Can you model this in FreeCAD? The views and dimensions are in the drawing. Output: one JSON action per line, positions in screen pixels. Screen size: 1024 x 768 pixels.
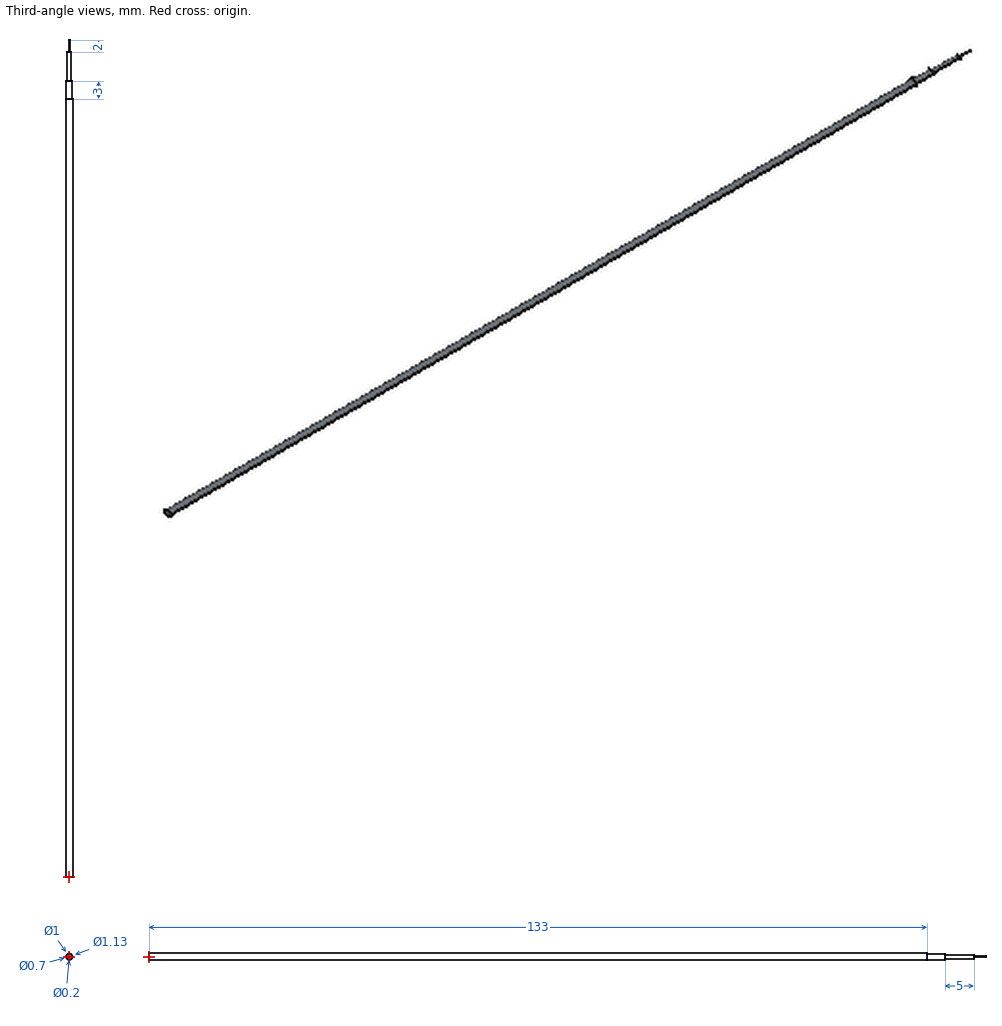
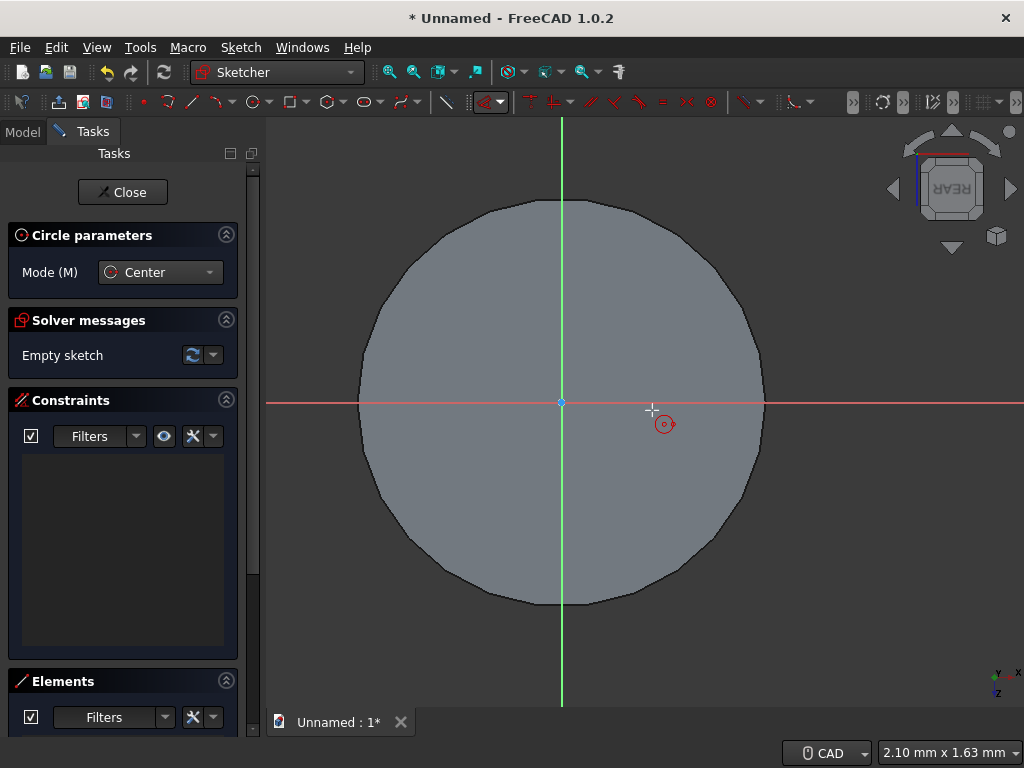
{"action": "left_click", "coordinate": [562, 403]}
{"action": "left_click", "coordinate": [689, 275]}
{"action": "key", "text": "Escape"}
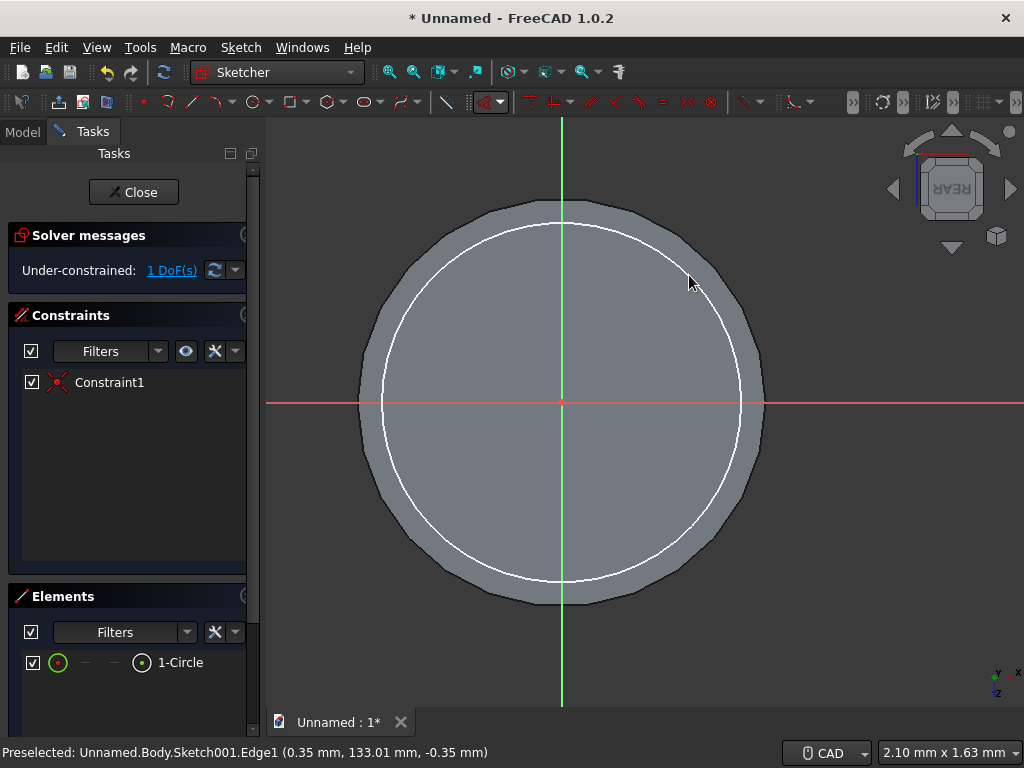
{"action": "left_click", "coordinate": [688, 275]}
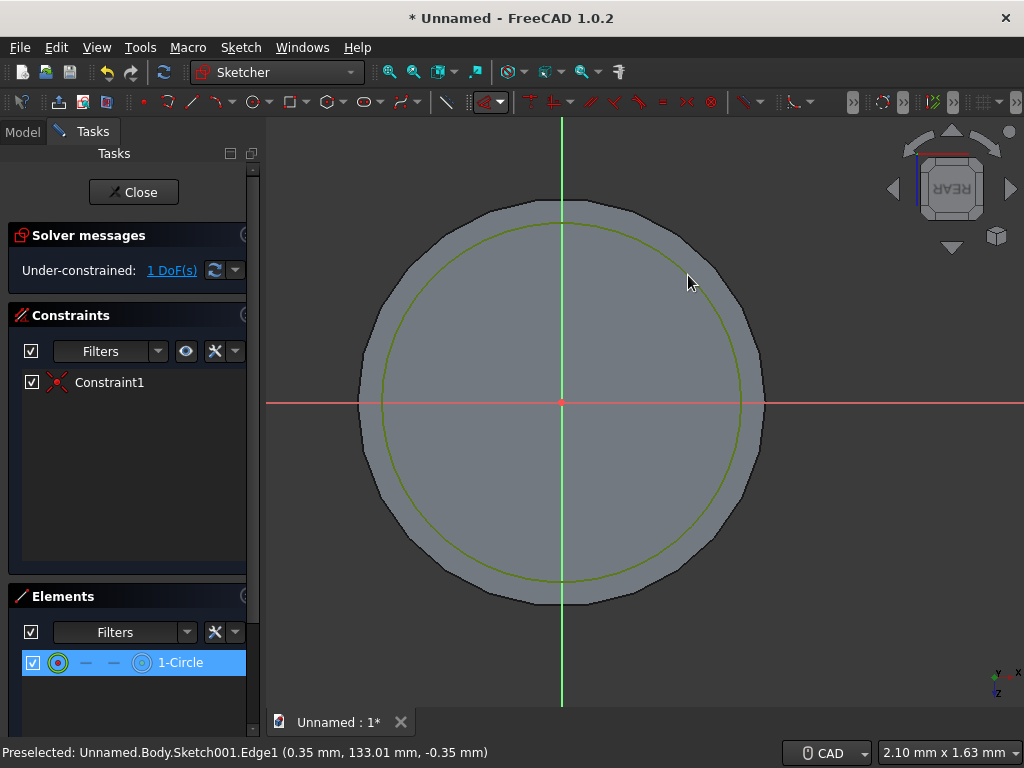
{"action": "left_click", "coordinate": [502, 102]}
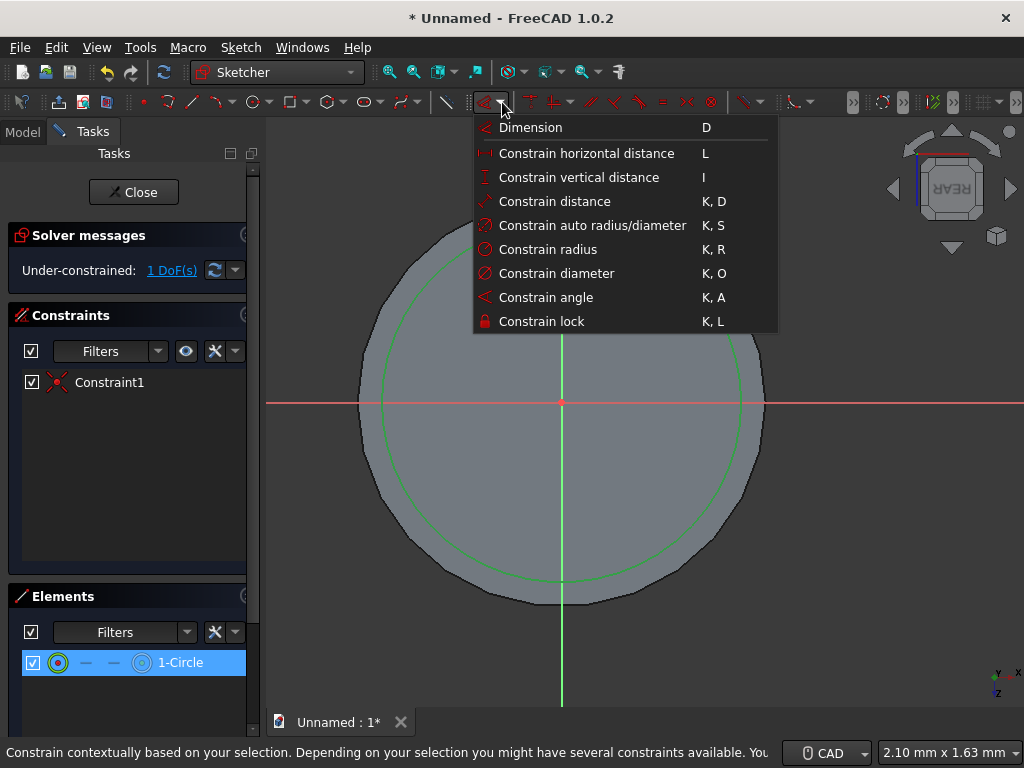
{"action": "left_click", "coordinate": [626, 273]}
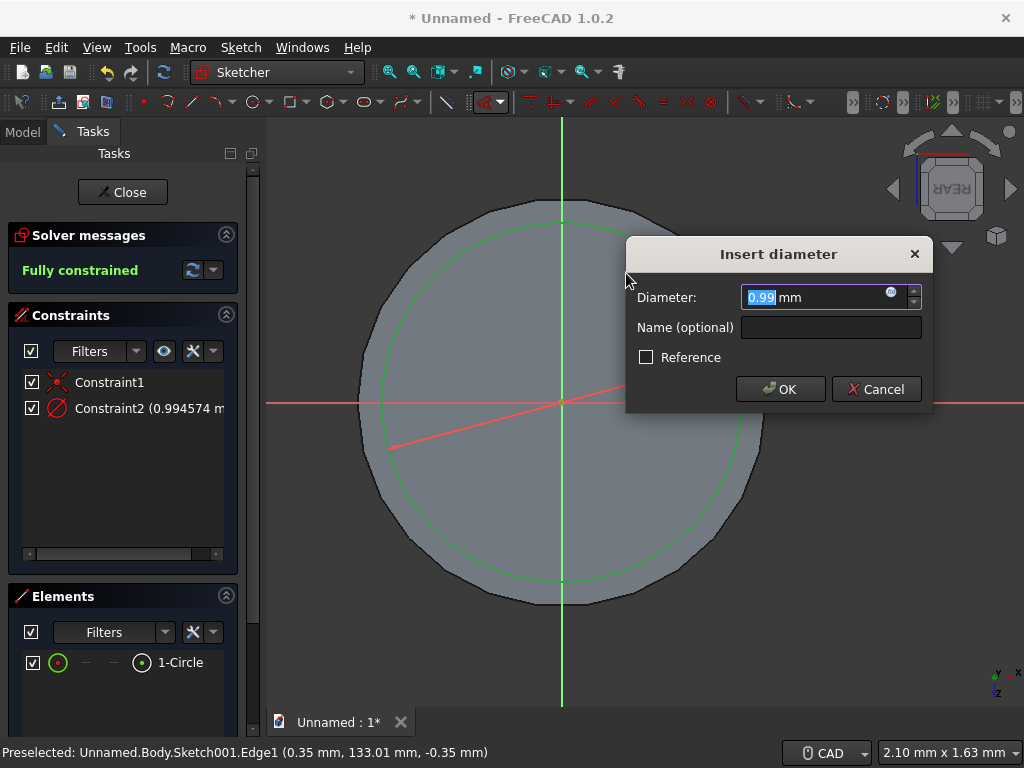
{"action": "type", "text": "1"}
{"action": "key", "text": "Return"}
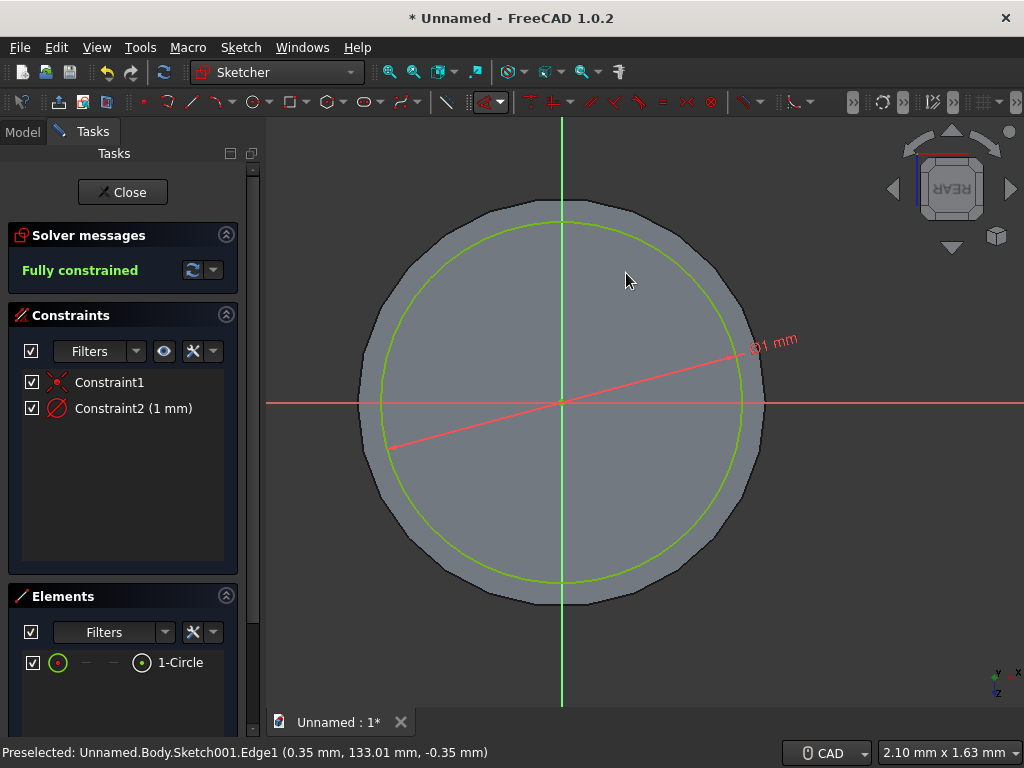
{"action": "left_click", "coordinate": [123, 192]}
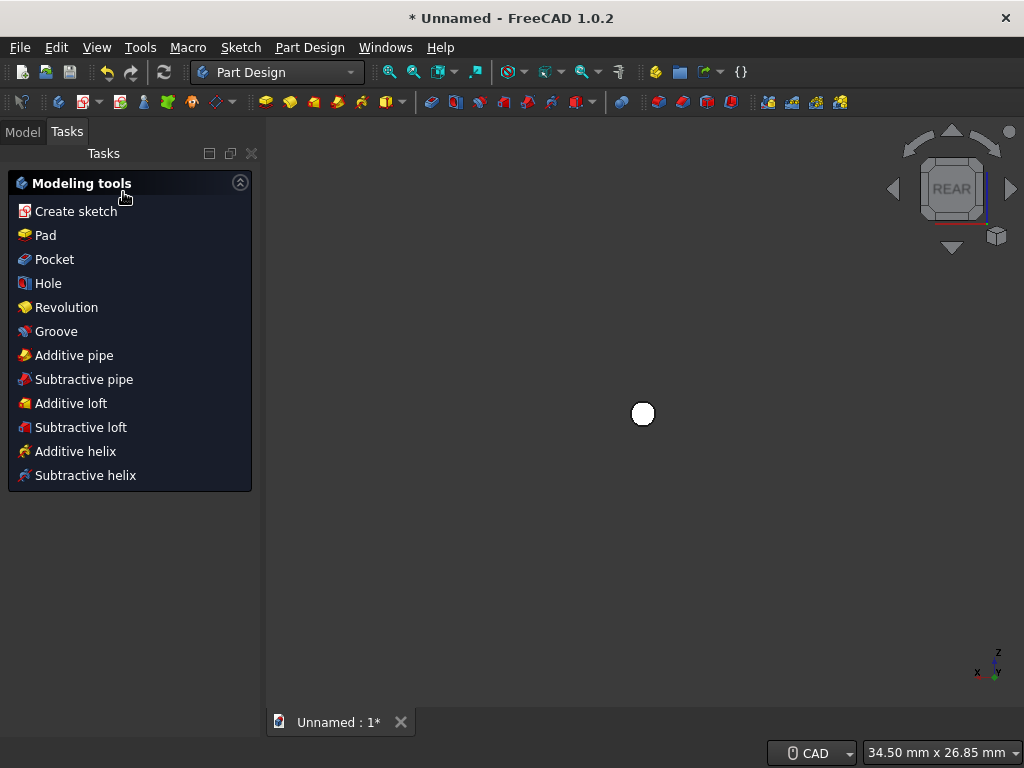
{"action": "left_click", "coordinate": [266, 102]}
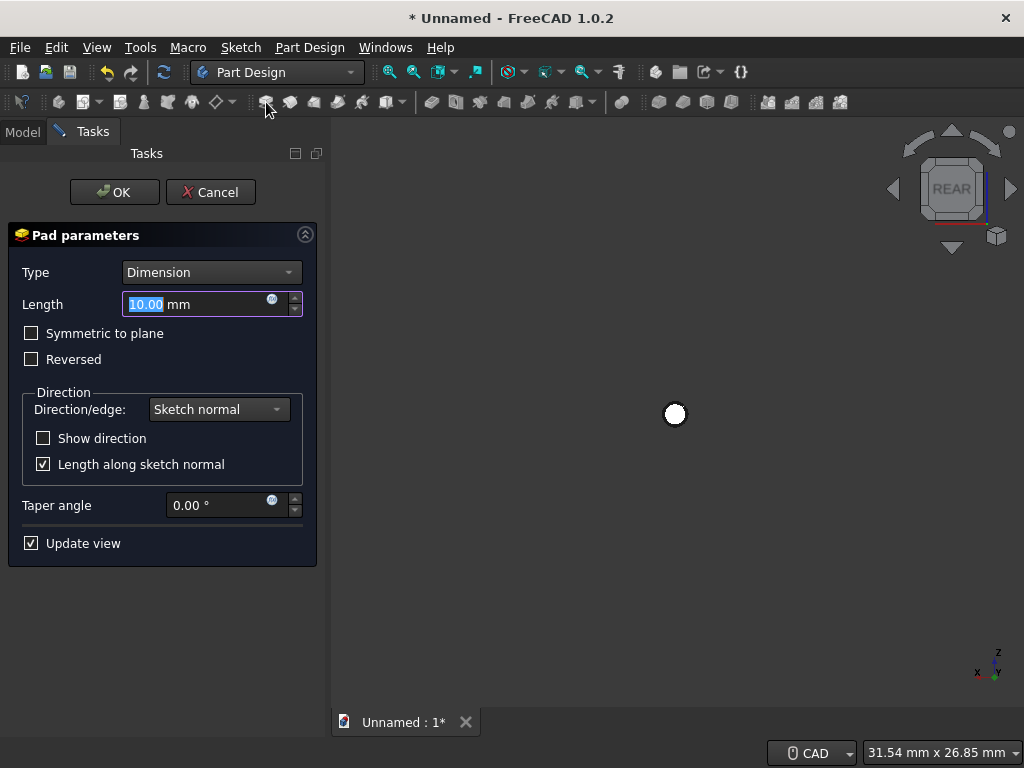
{"action": "type", "text": "3"}
{"action": "key", "text": "Tab"}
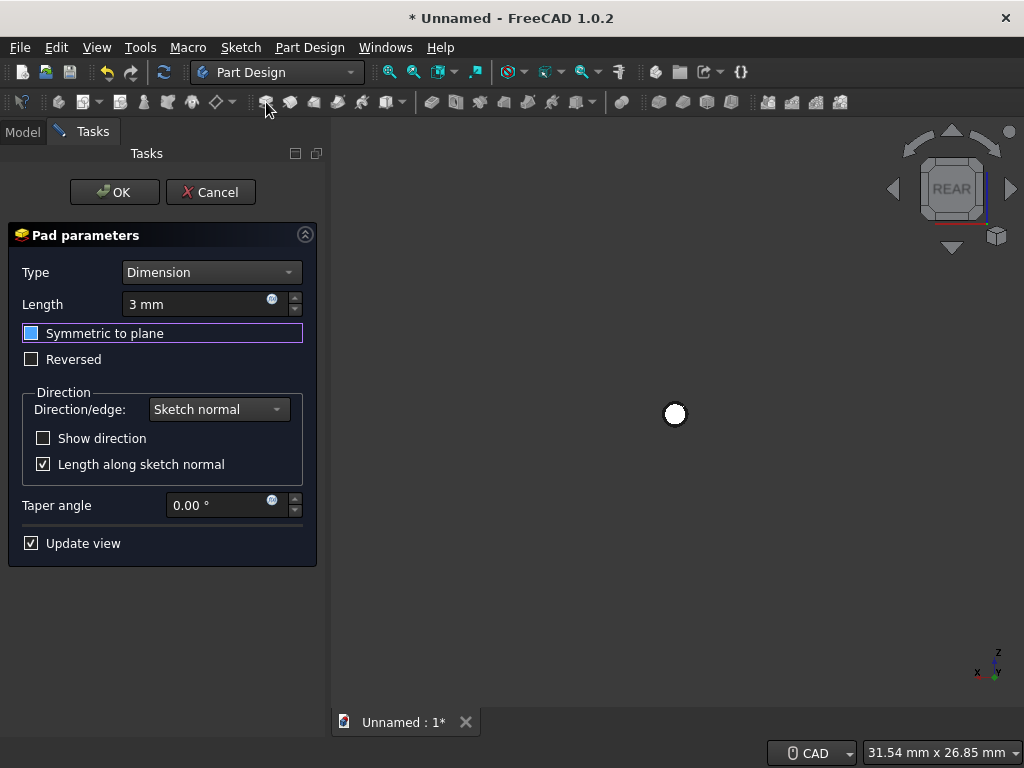
{"action": "left_click", "coordinate": [115, 192]}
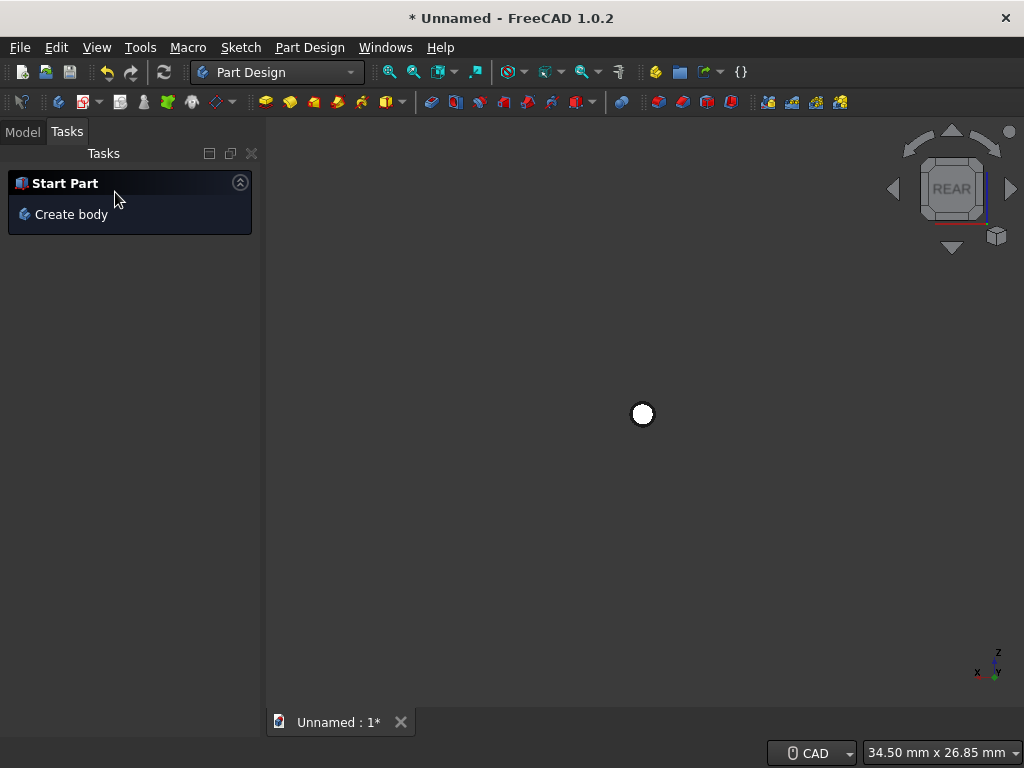
{"action": "left_click", "coordinate": [390, 72]}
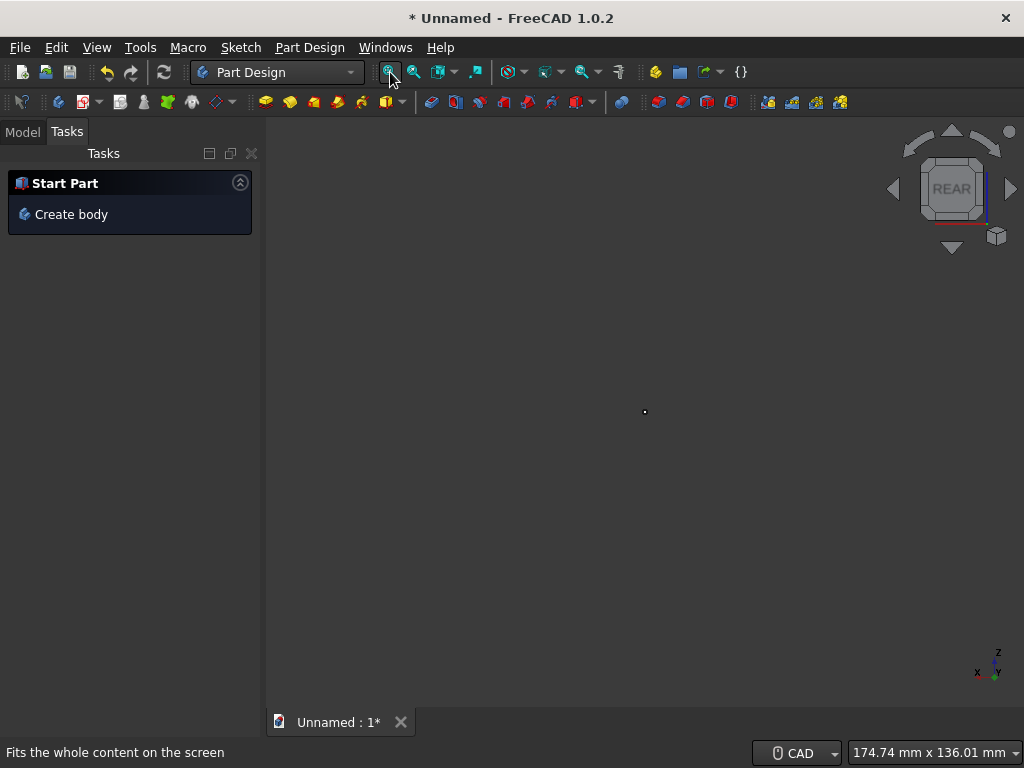
{"action": "scroll", "coordinate": [645, 411], "scroll_direction": "up", "scroll_amount": 9}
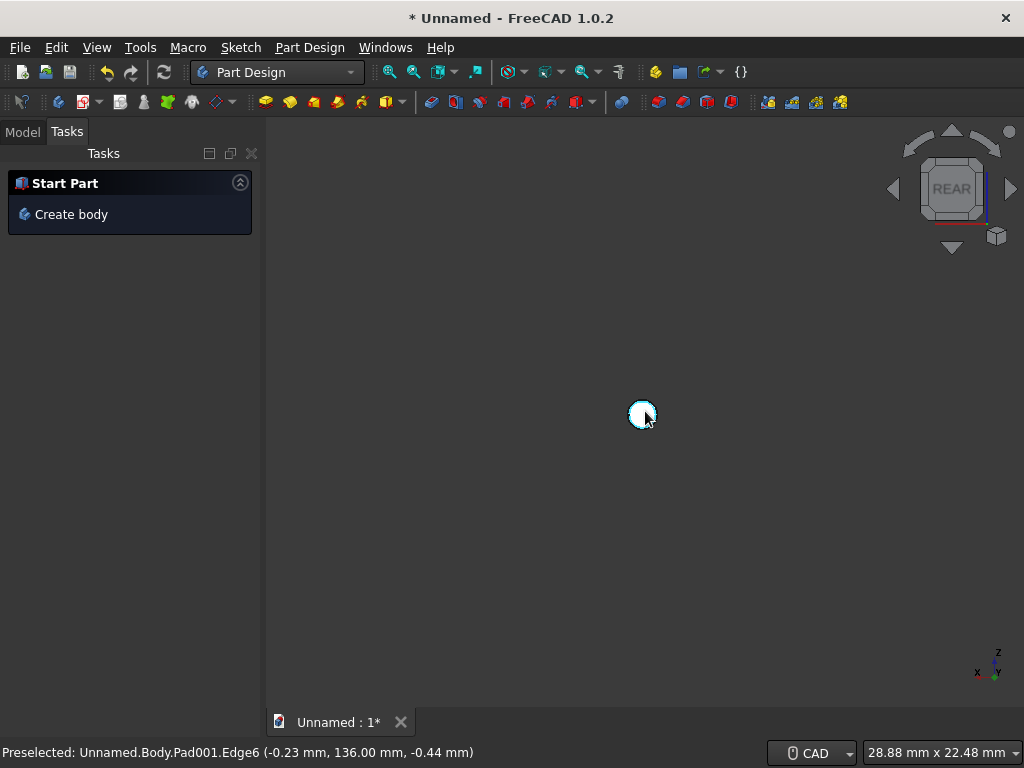
{"action": "left_click", "coordinate": [642, 414]}